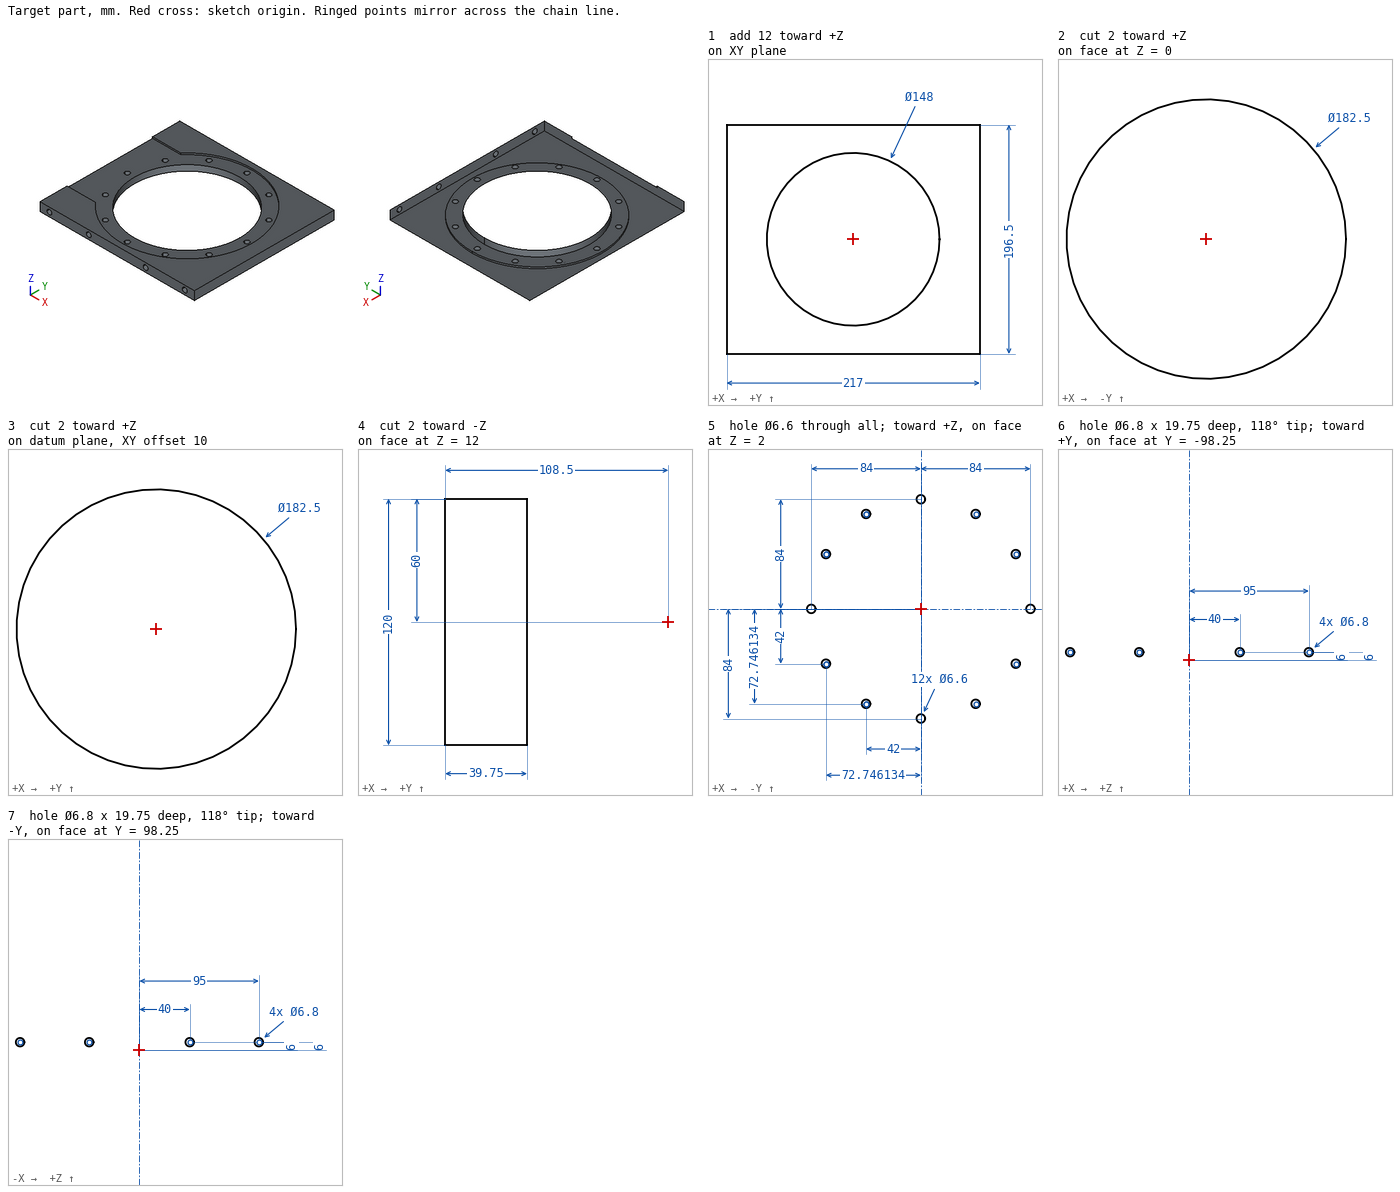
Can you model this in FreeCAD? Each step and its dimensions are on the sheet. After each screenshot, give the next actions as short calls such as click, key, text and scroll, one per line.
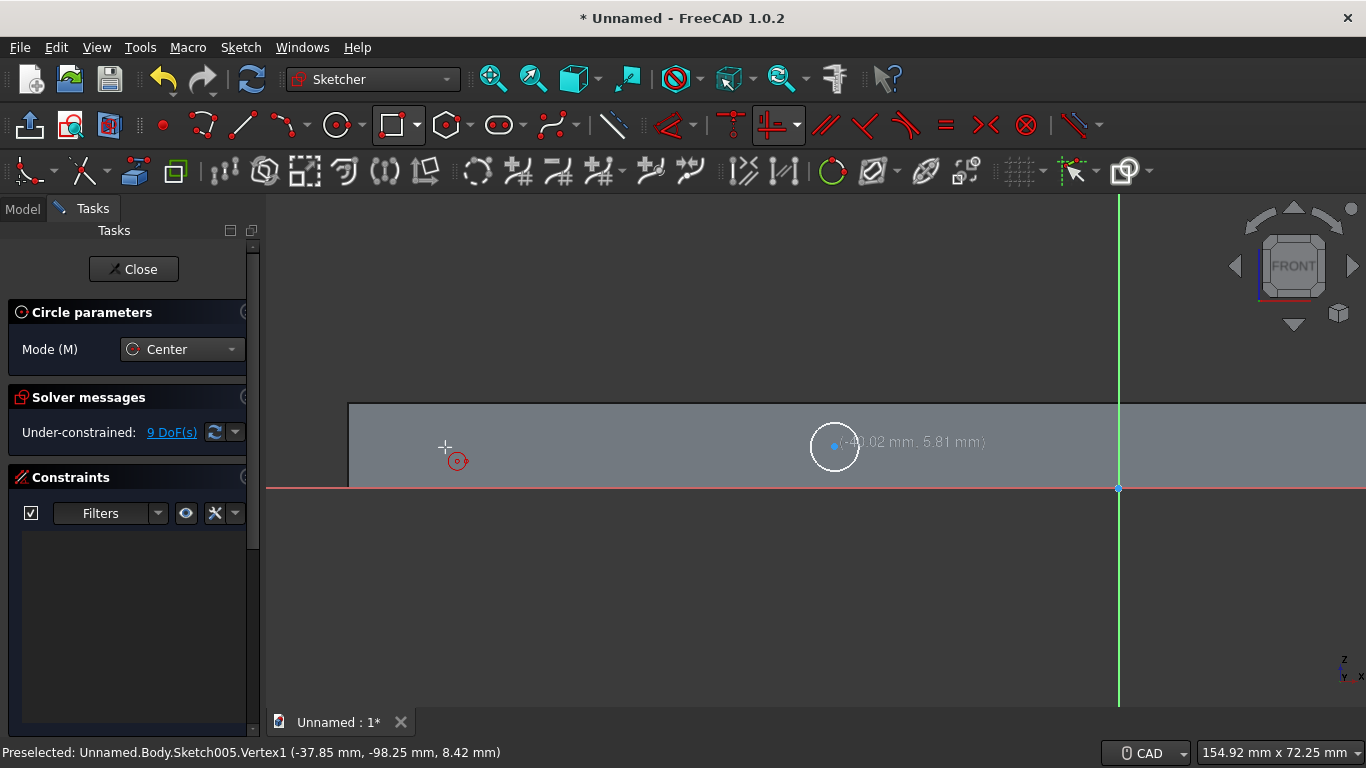
click(444, 446)
click(461, 429)
key(Escape)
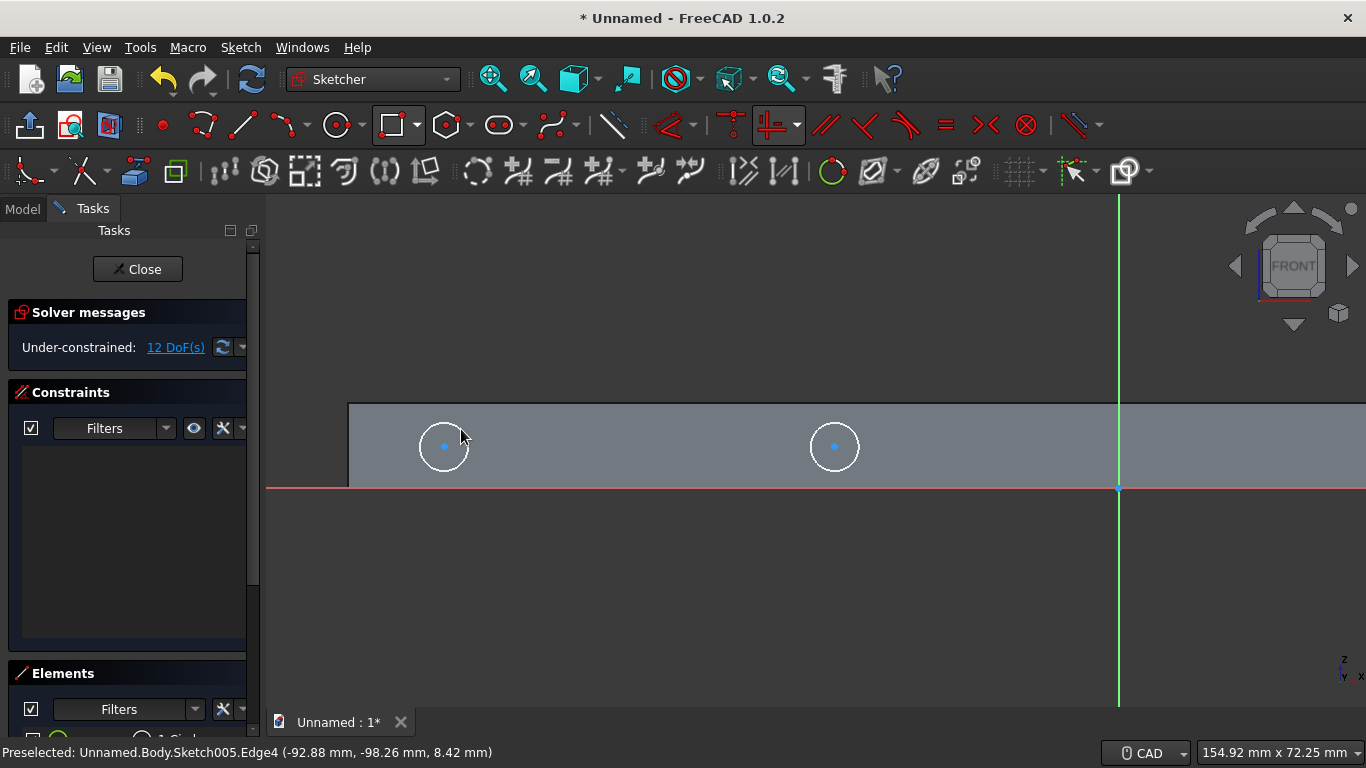
scroll(445, 447, down, 4)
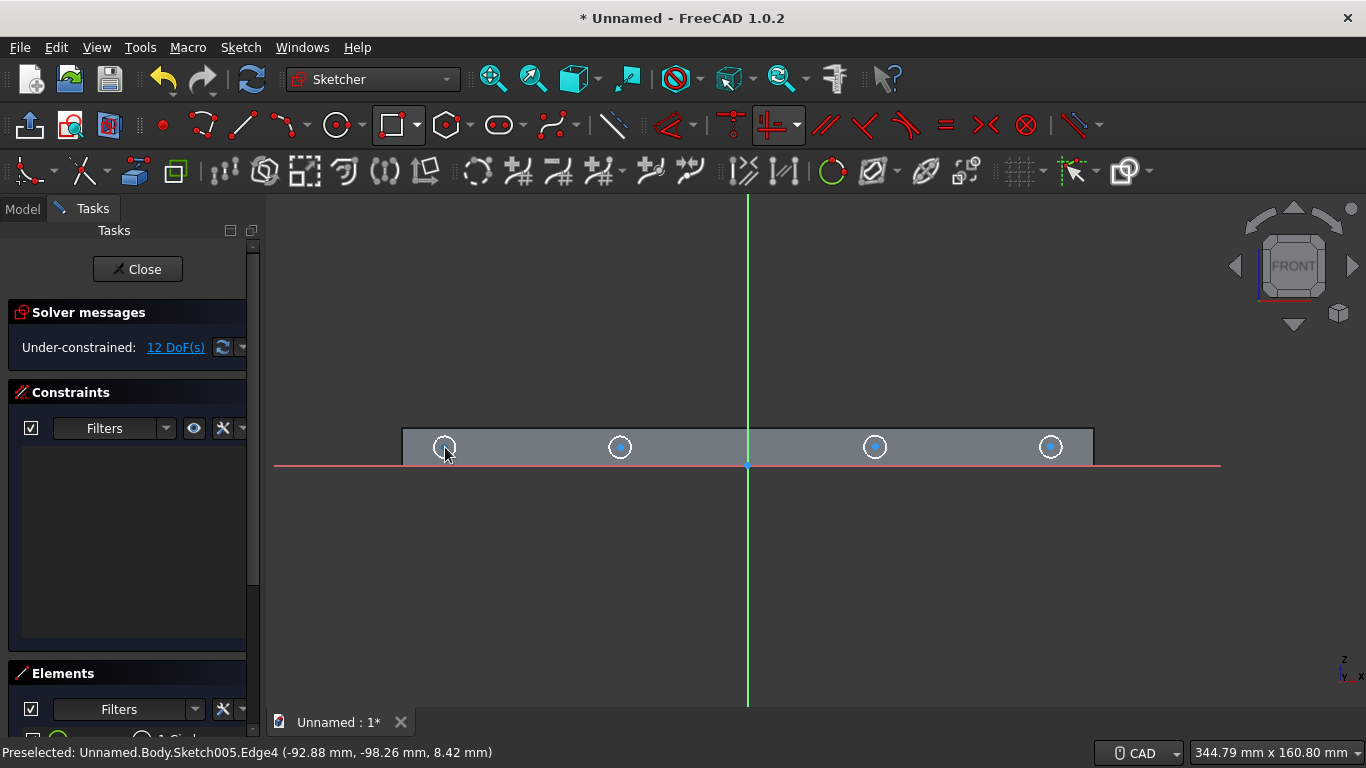
scroll(1059, 439, up, 2)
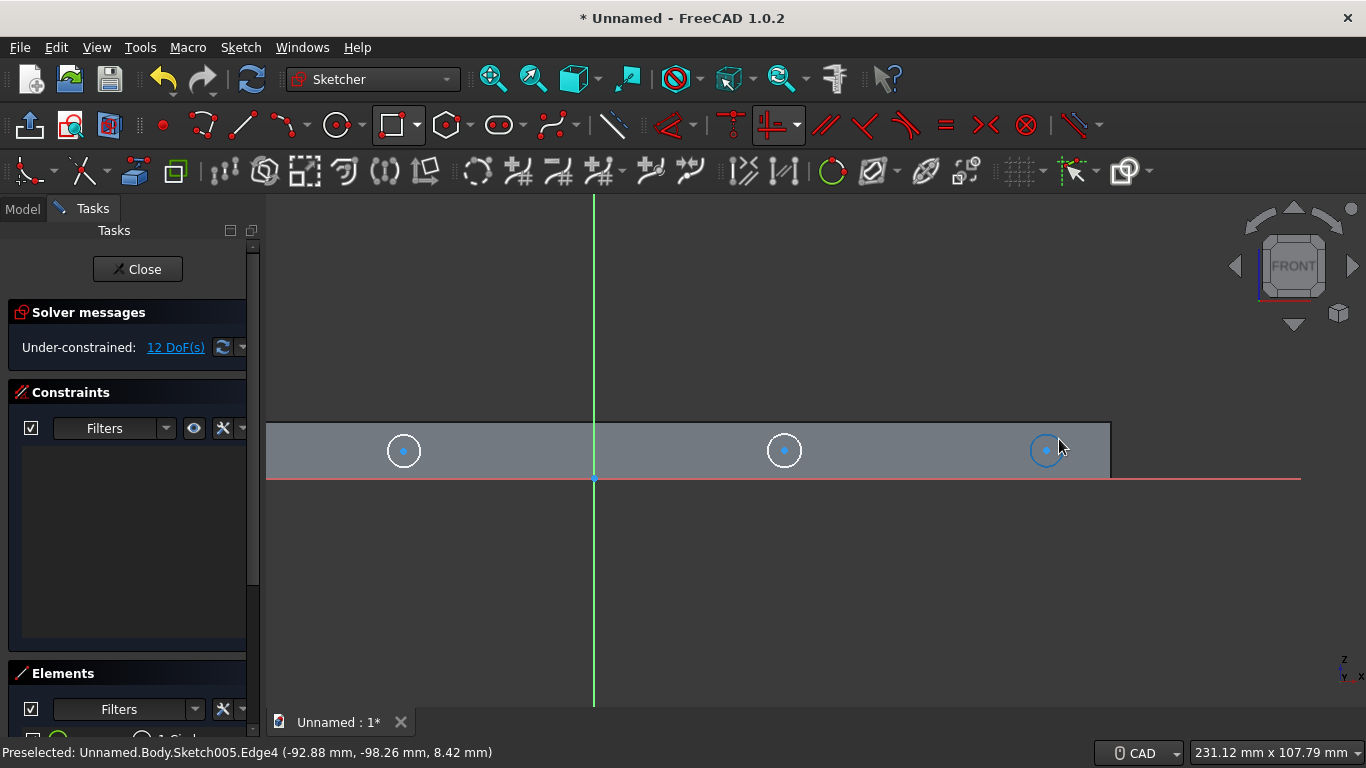
click(1058, 439)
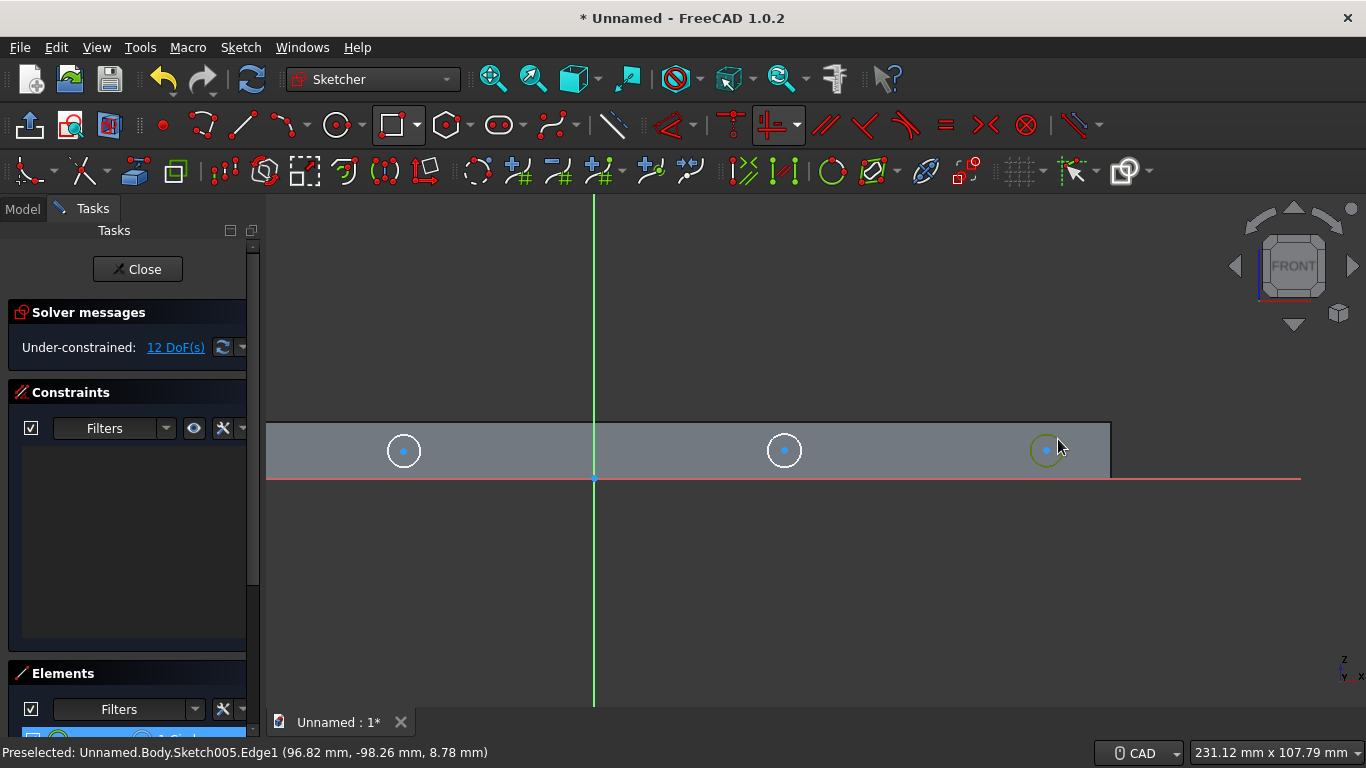
click(796, 439)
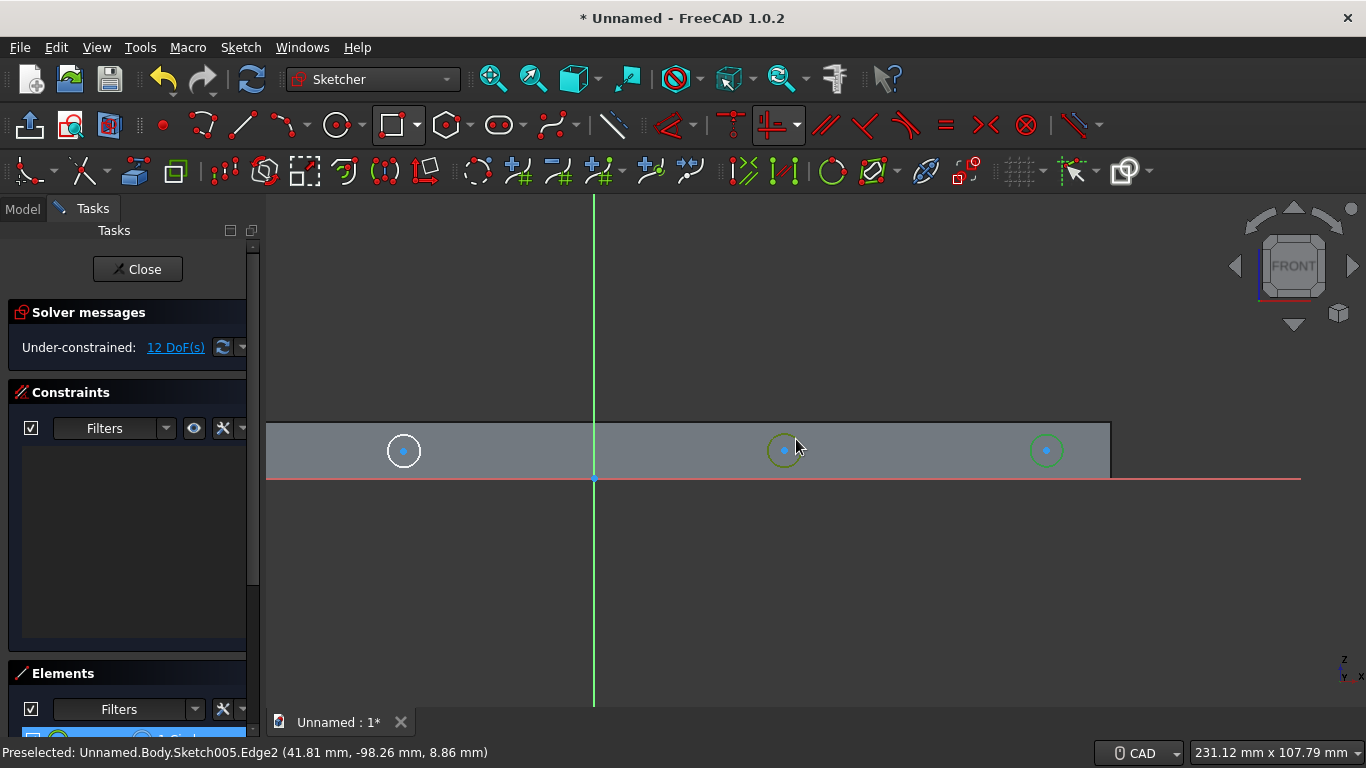
click(415, 440)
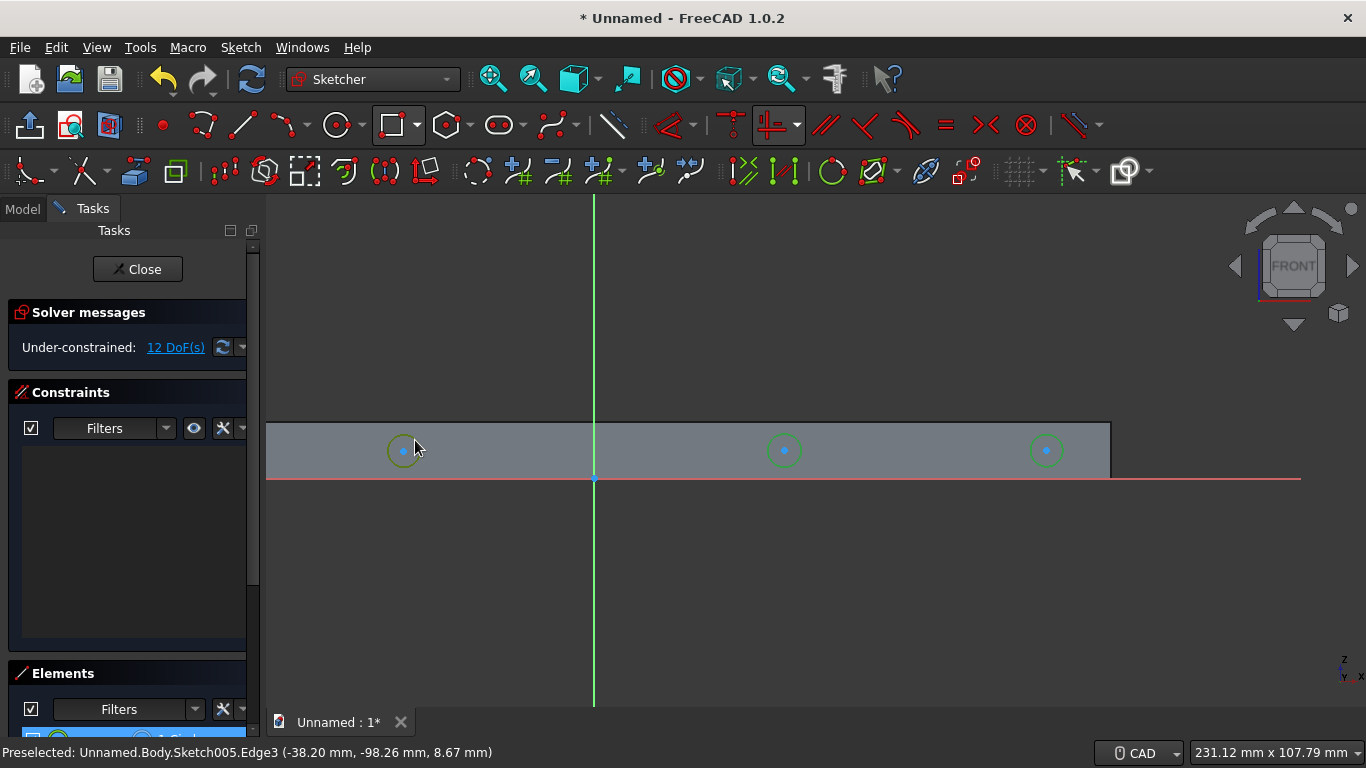
scroll(1059, 439, down, 2)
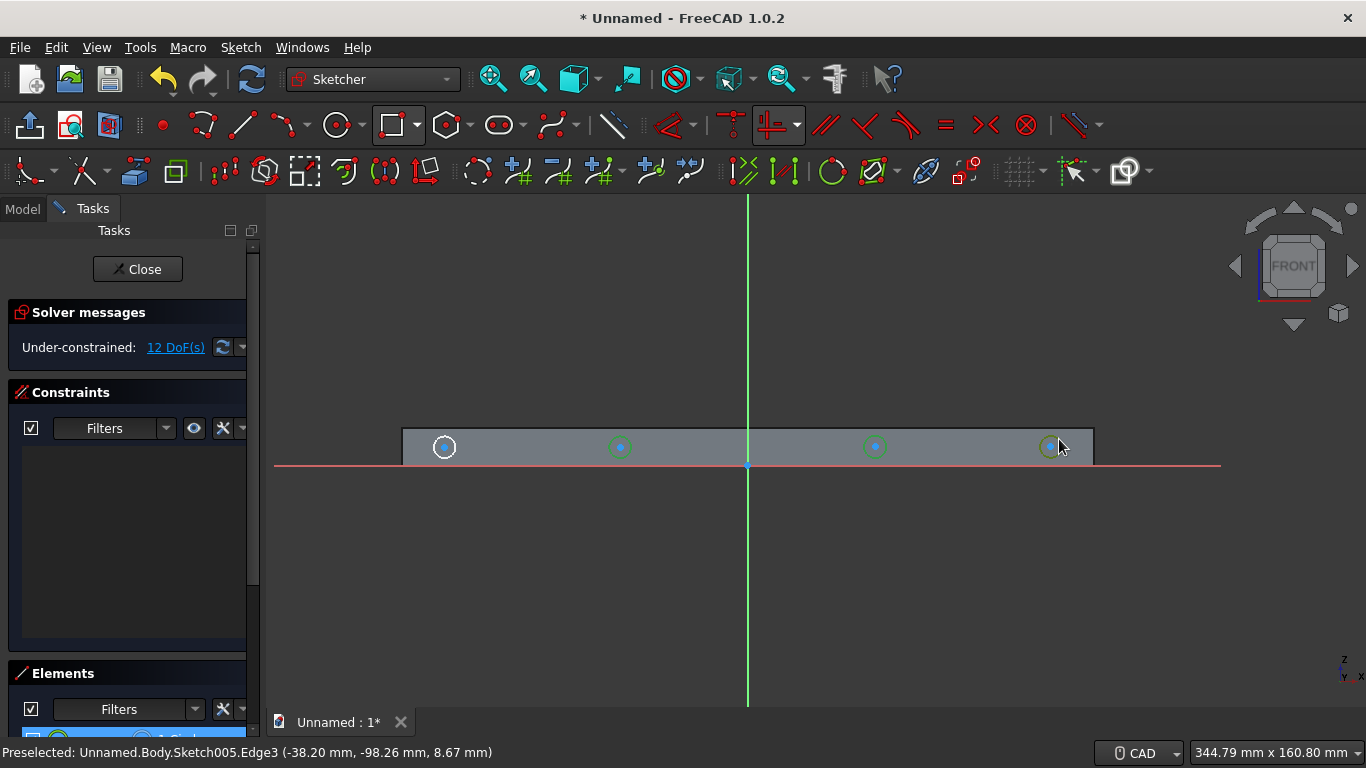
scroll(452, 440, up, 2)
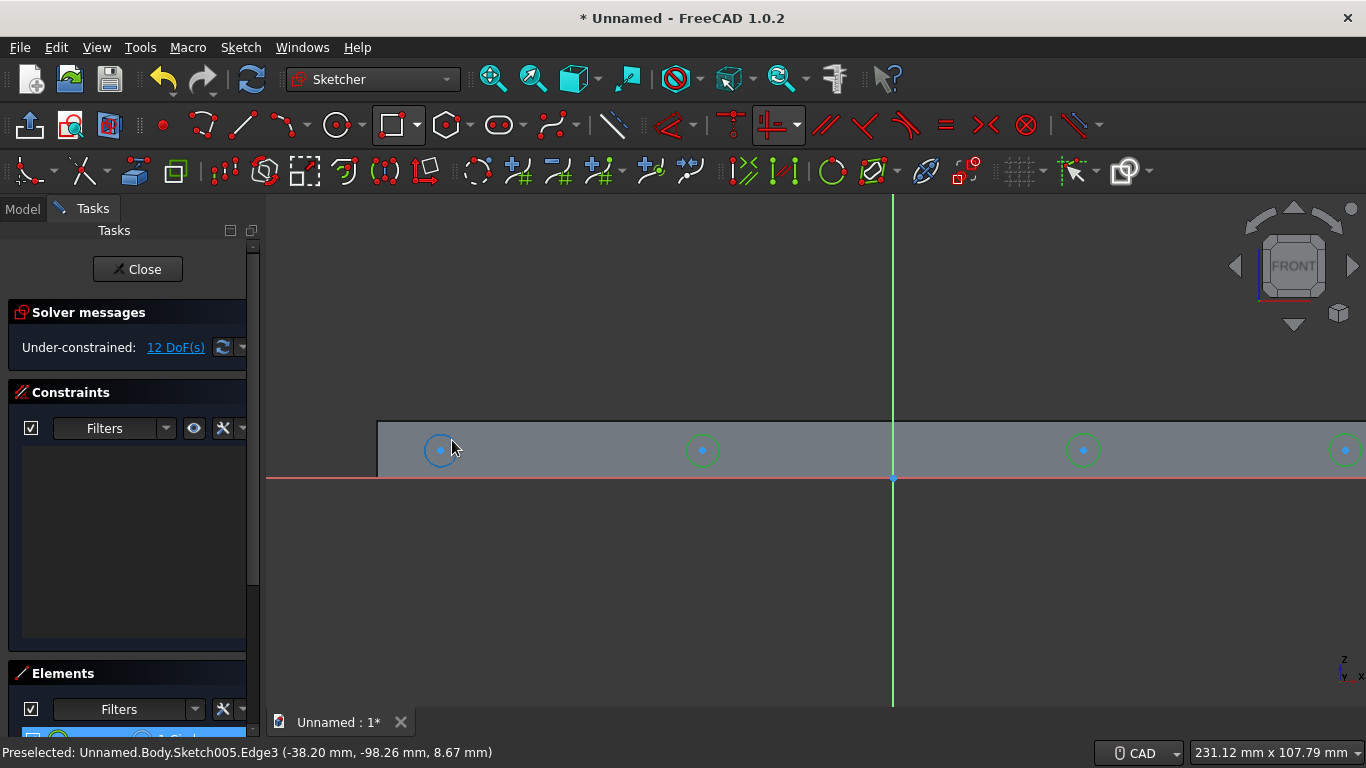
click(452, 439)